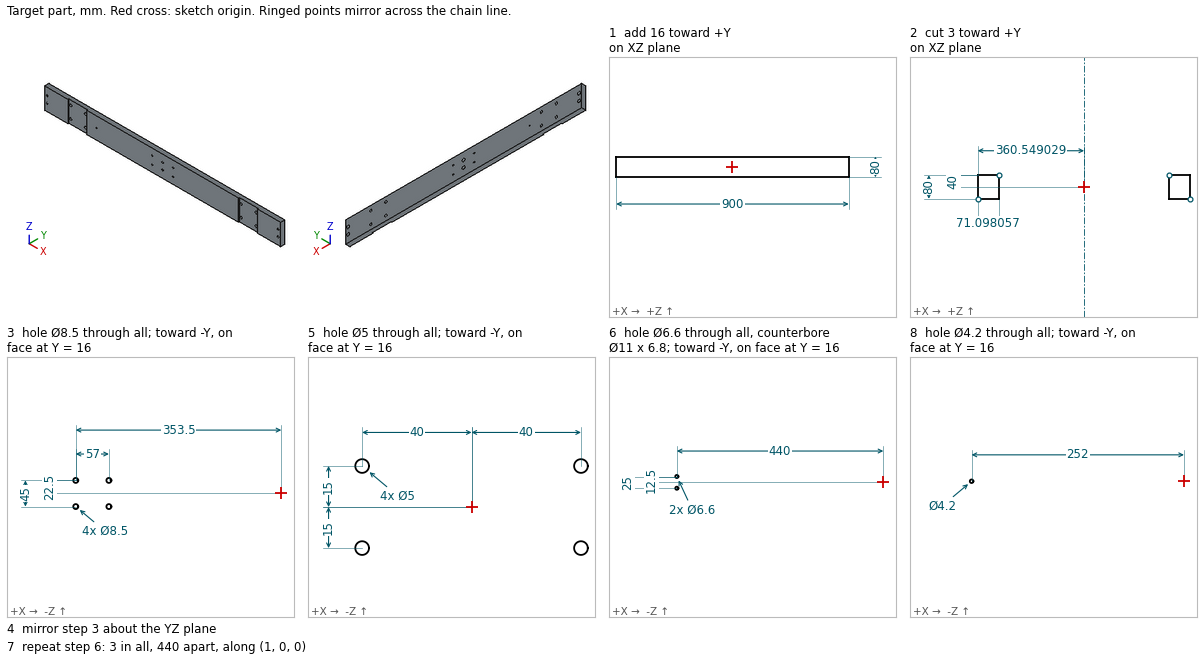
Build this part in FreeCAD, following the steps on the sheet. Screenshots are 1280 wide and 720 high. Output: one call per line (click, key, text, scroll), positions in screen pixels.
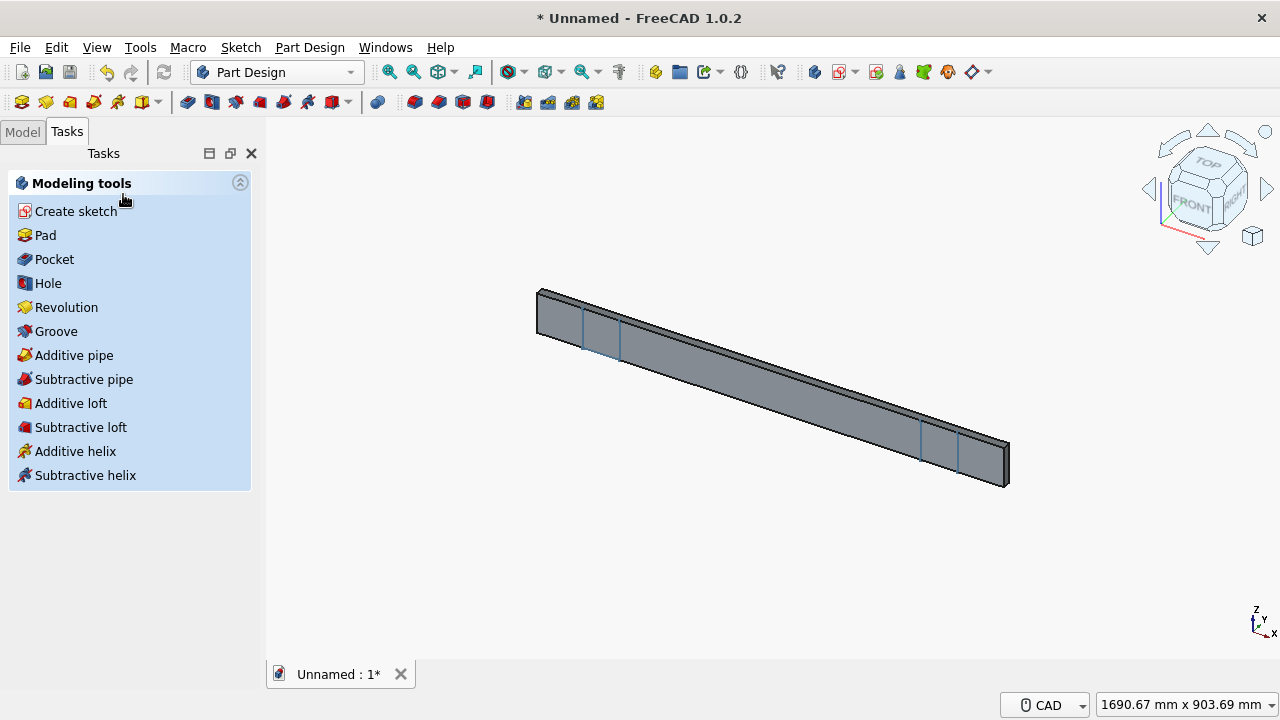
click(188, 102)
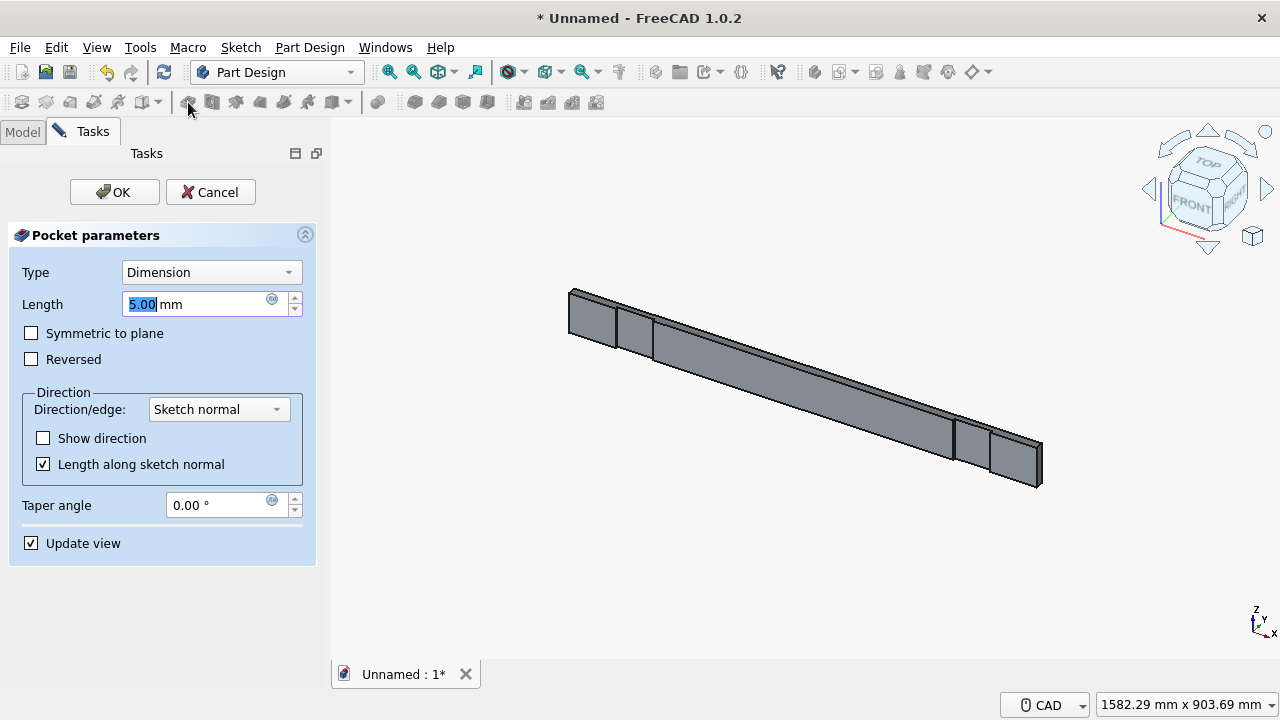
text(3)
key(Tab)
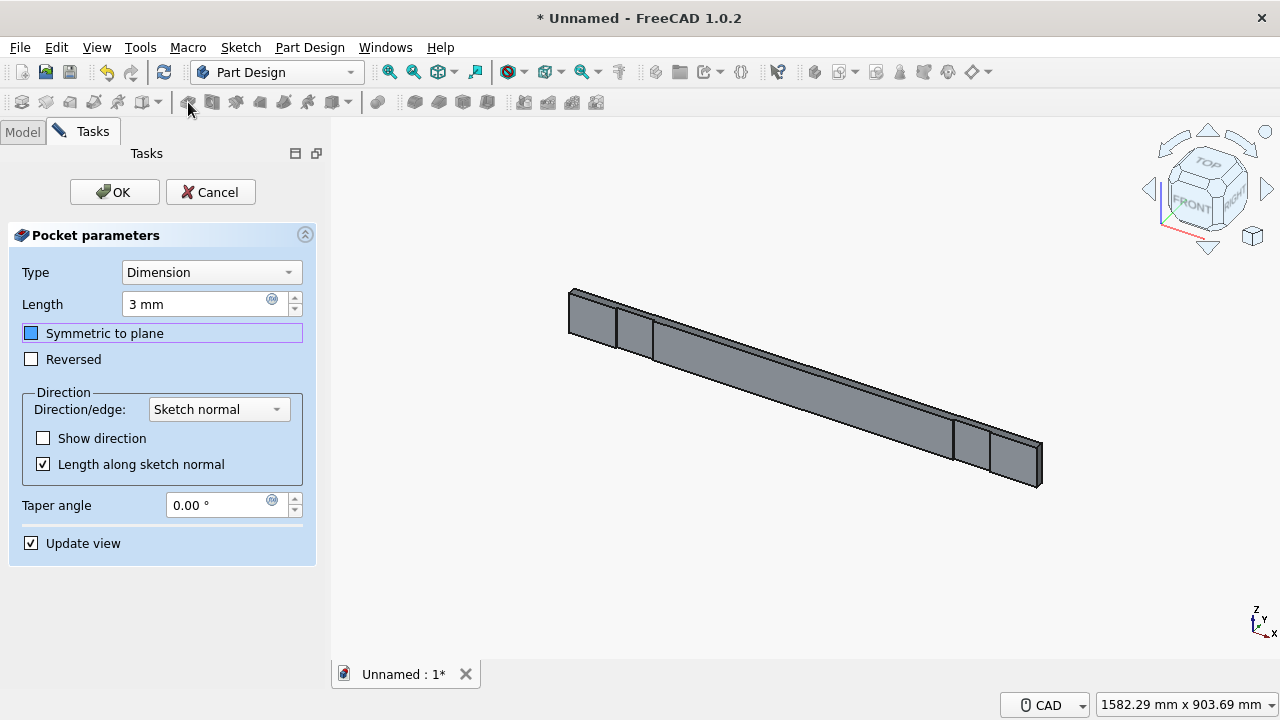
click(115, 192)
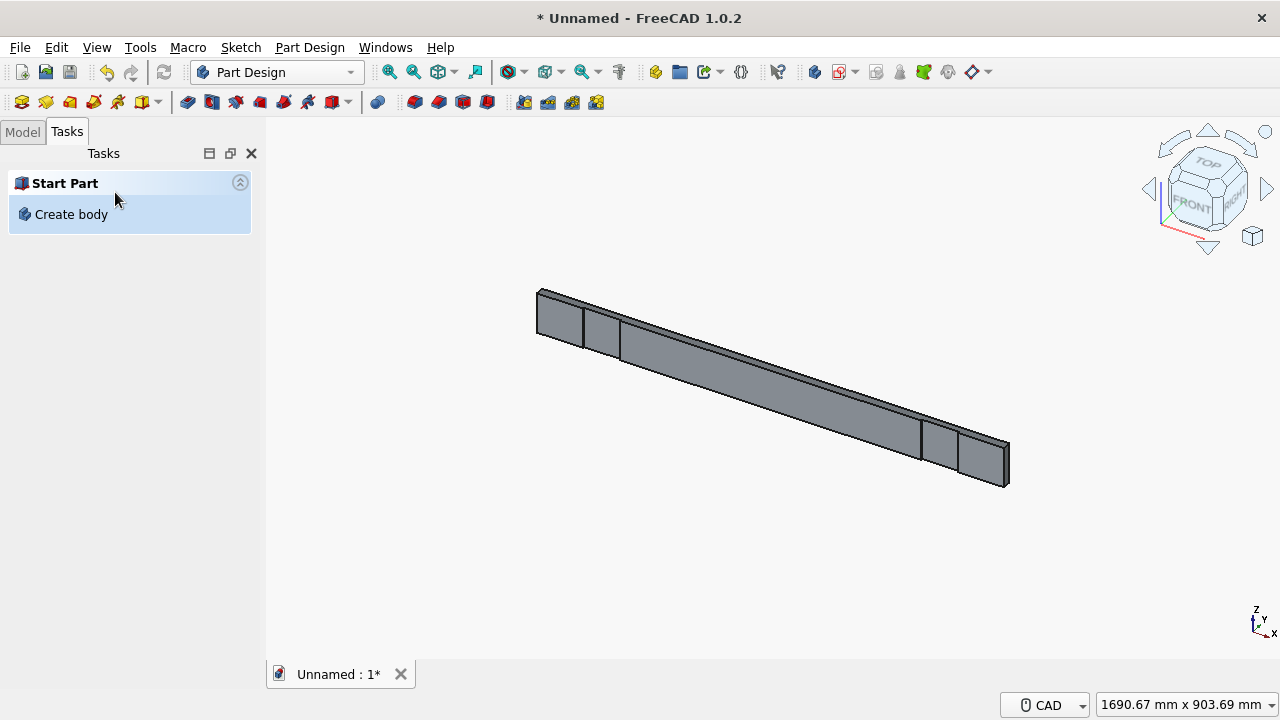
key(4)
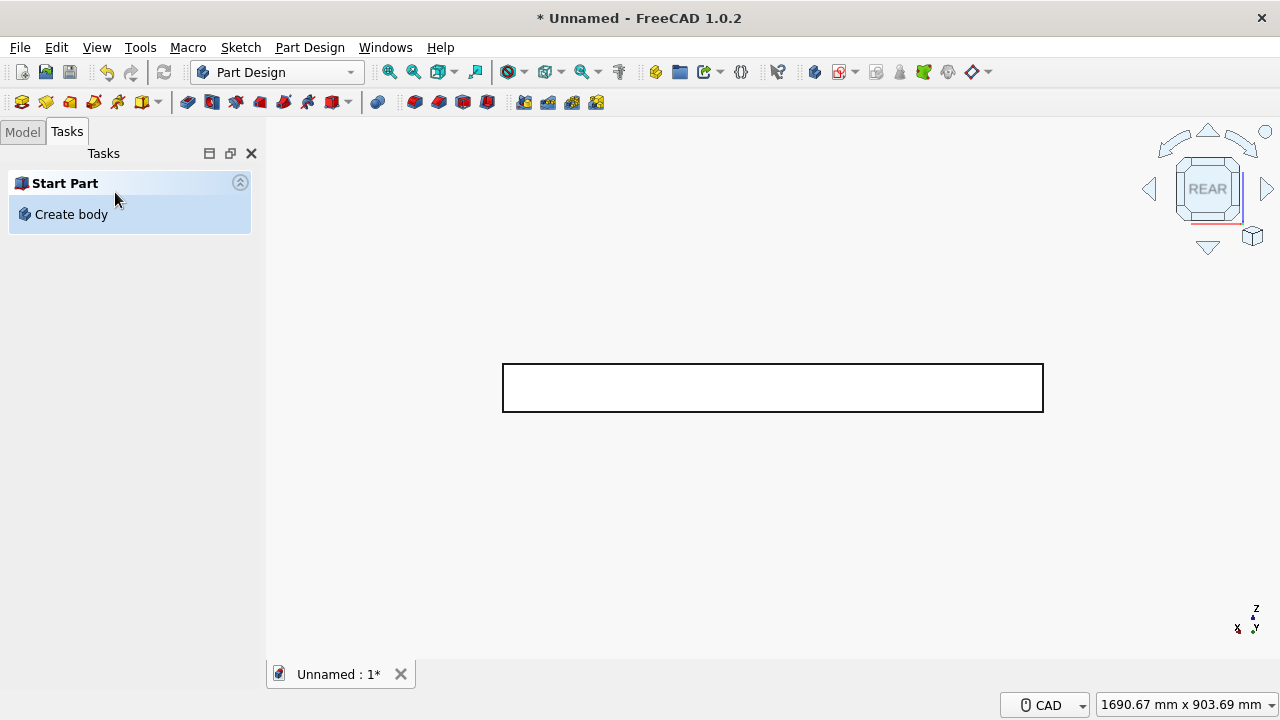
click(542, 387)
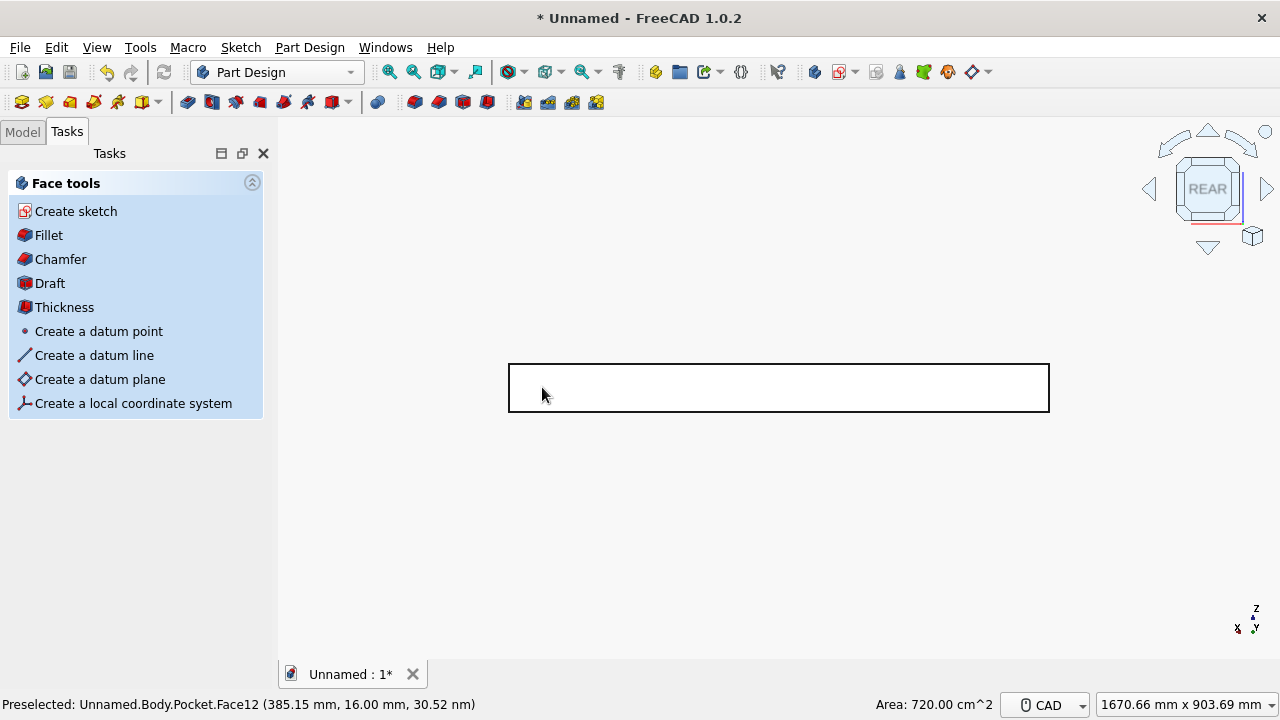
click(840, 72)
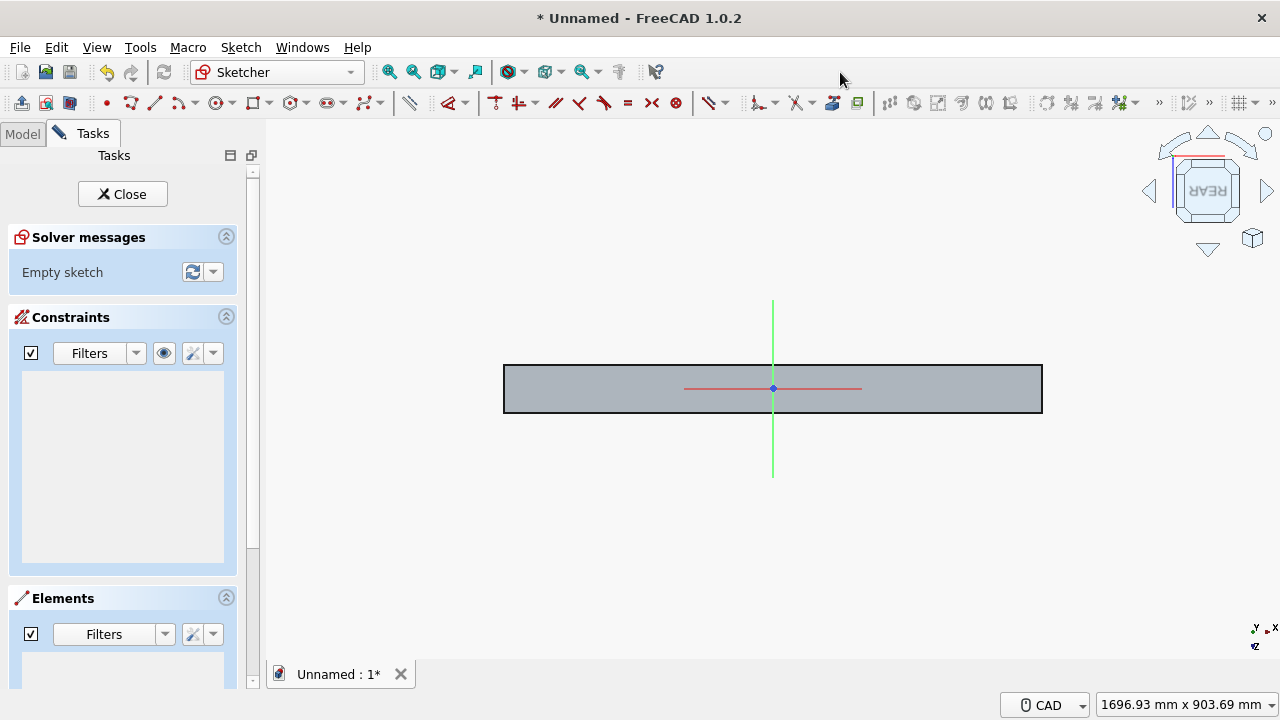
scroll(566, 389, up, 12)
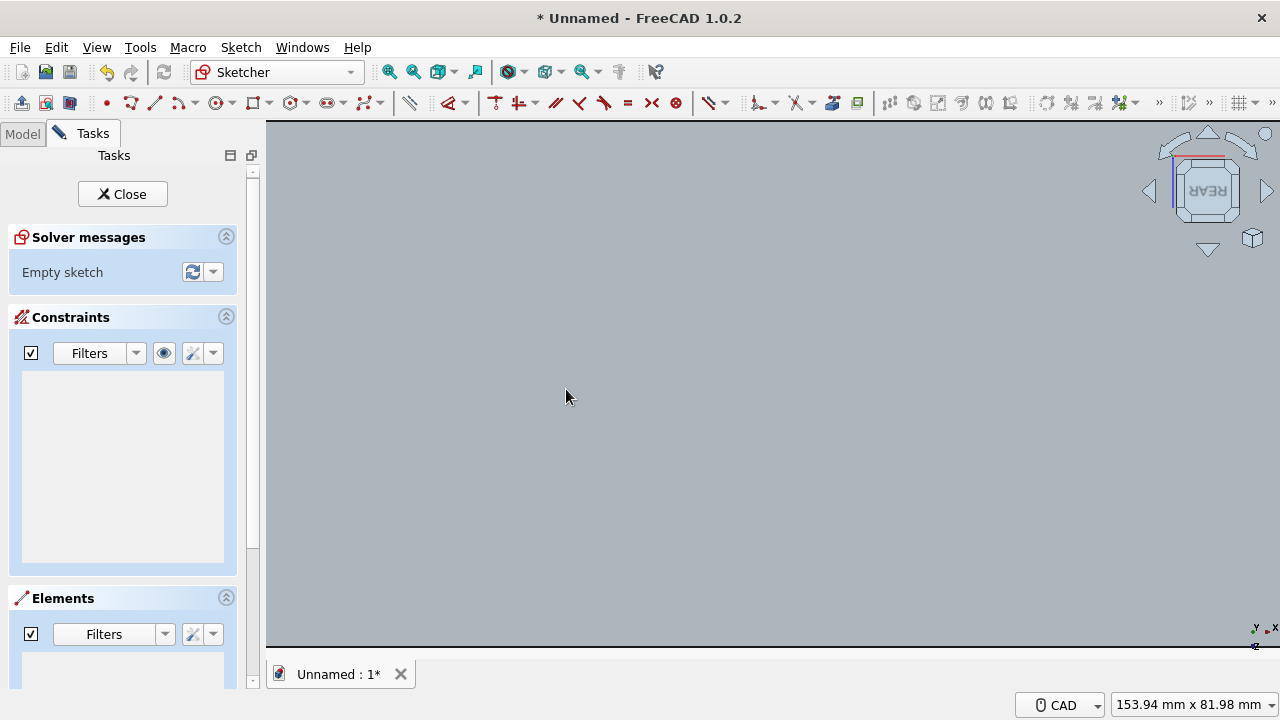
click(216, 104)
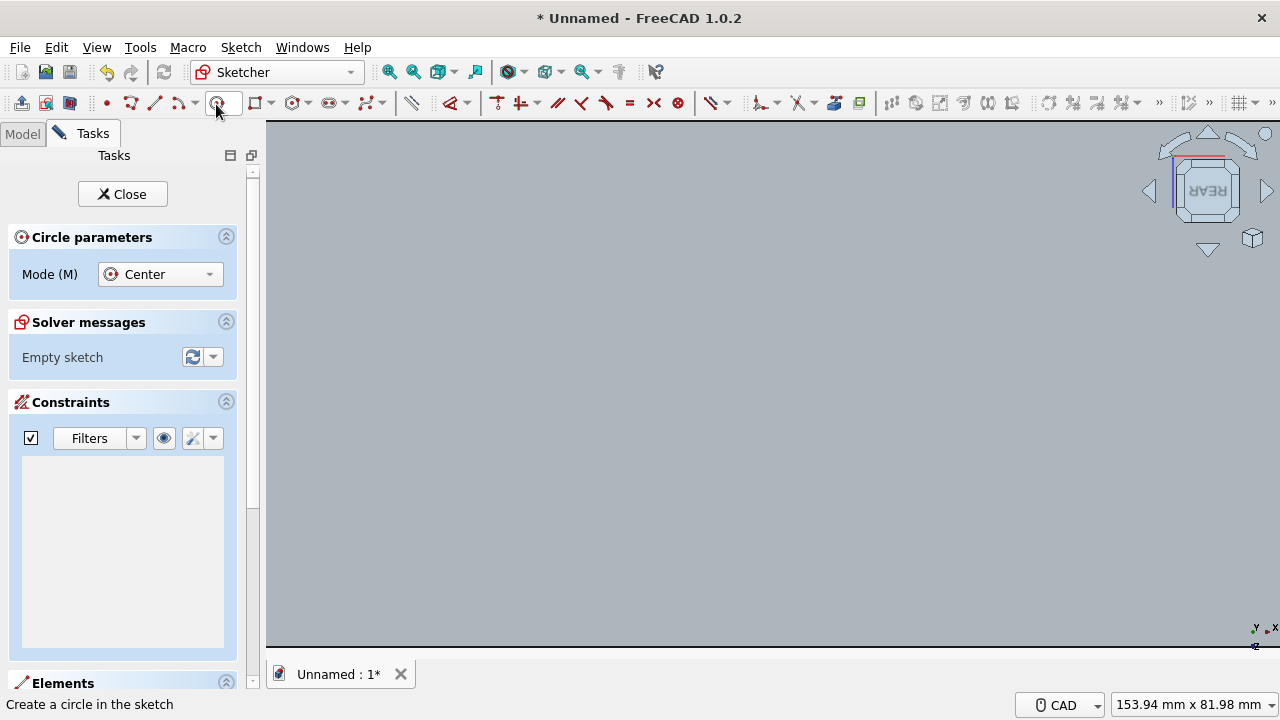
click(516, 236)
click(536, 216)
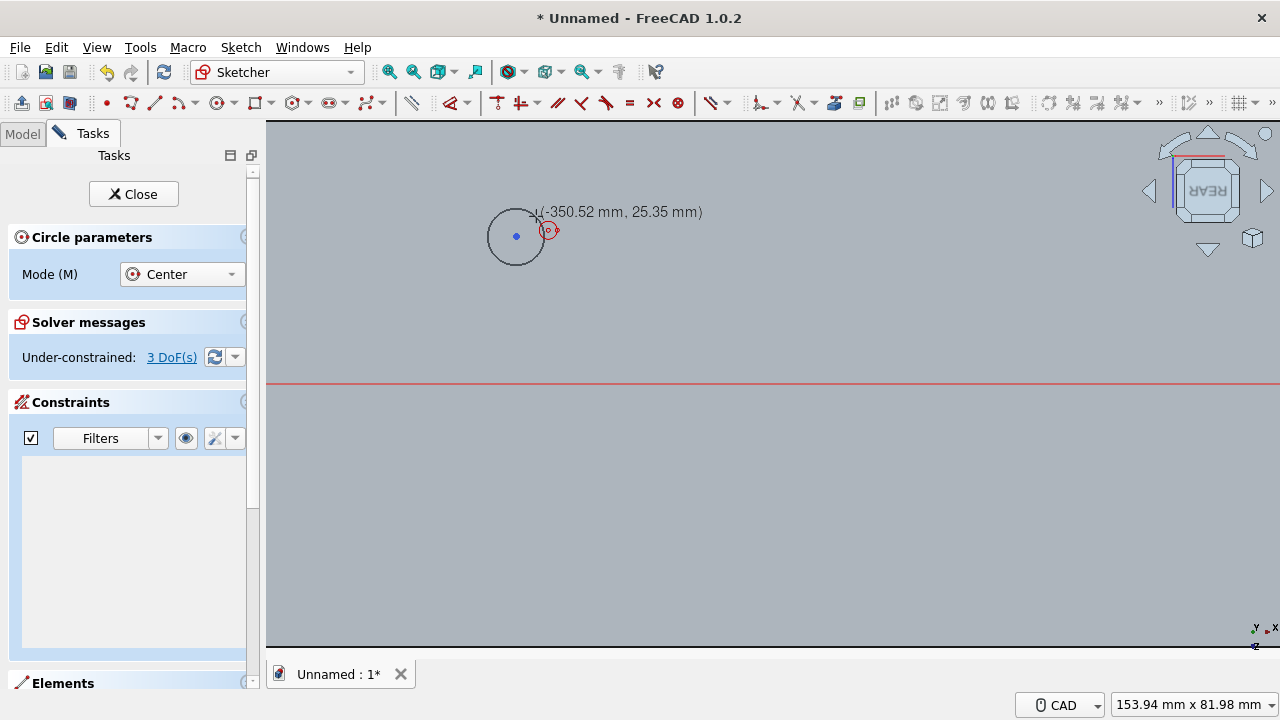
click(892, 236)
click(912, 216)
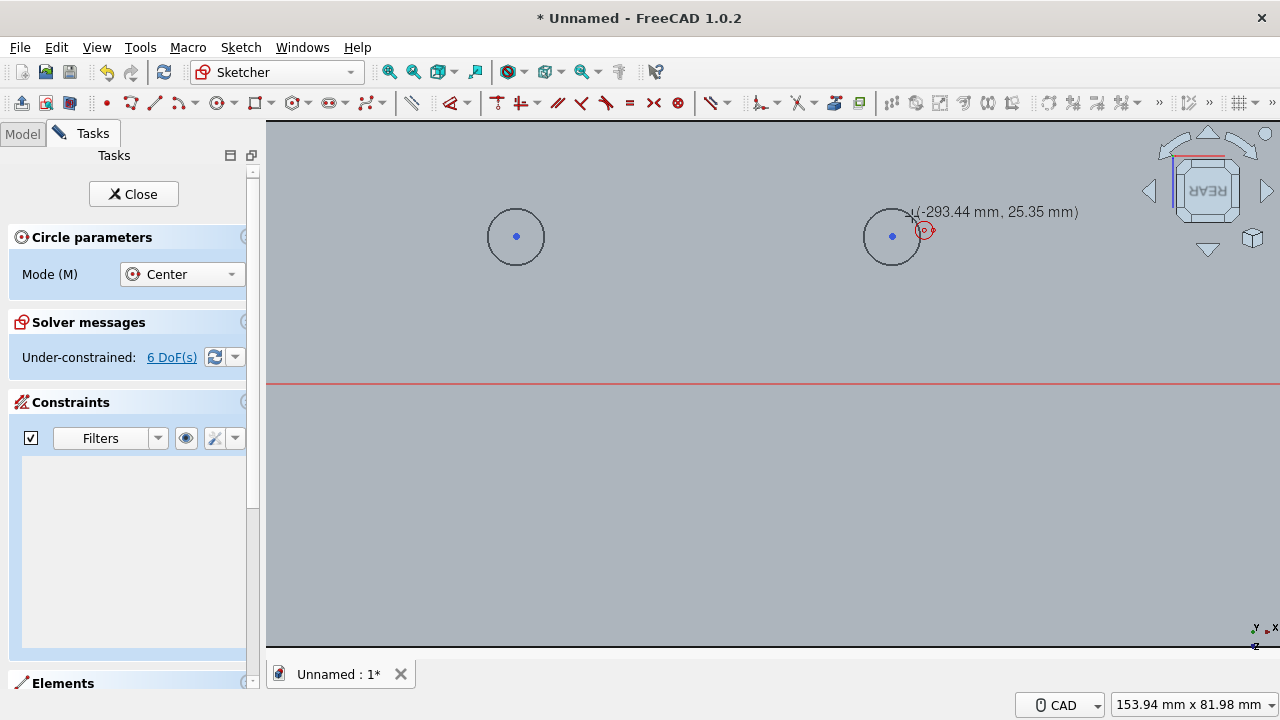
click(516, 532)
click(536, 512)